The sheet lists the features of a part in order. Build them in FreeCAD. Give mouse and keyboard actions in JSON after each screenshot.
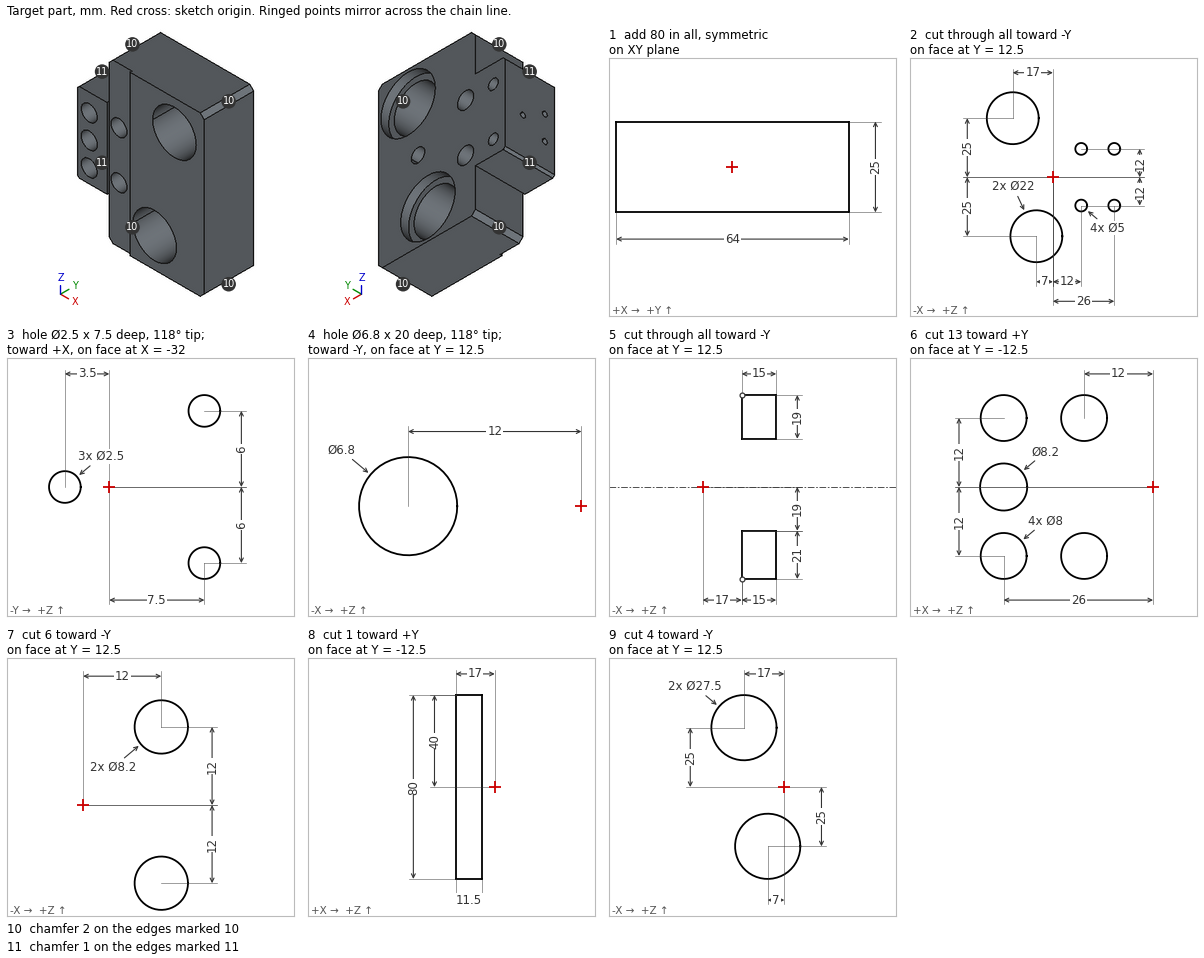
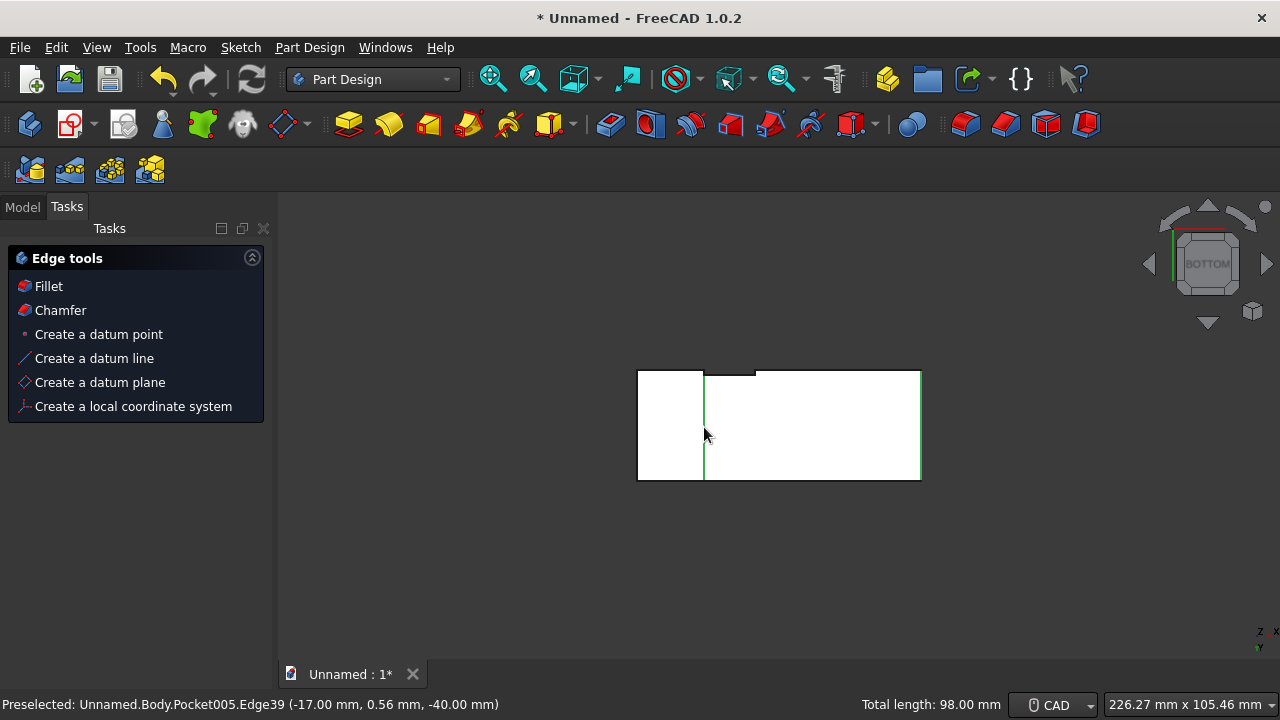
{"action": "left_click", "coordinate": [1006, 124]}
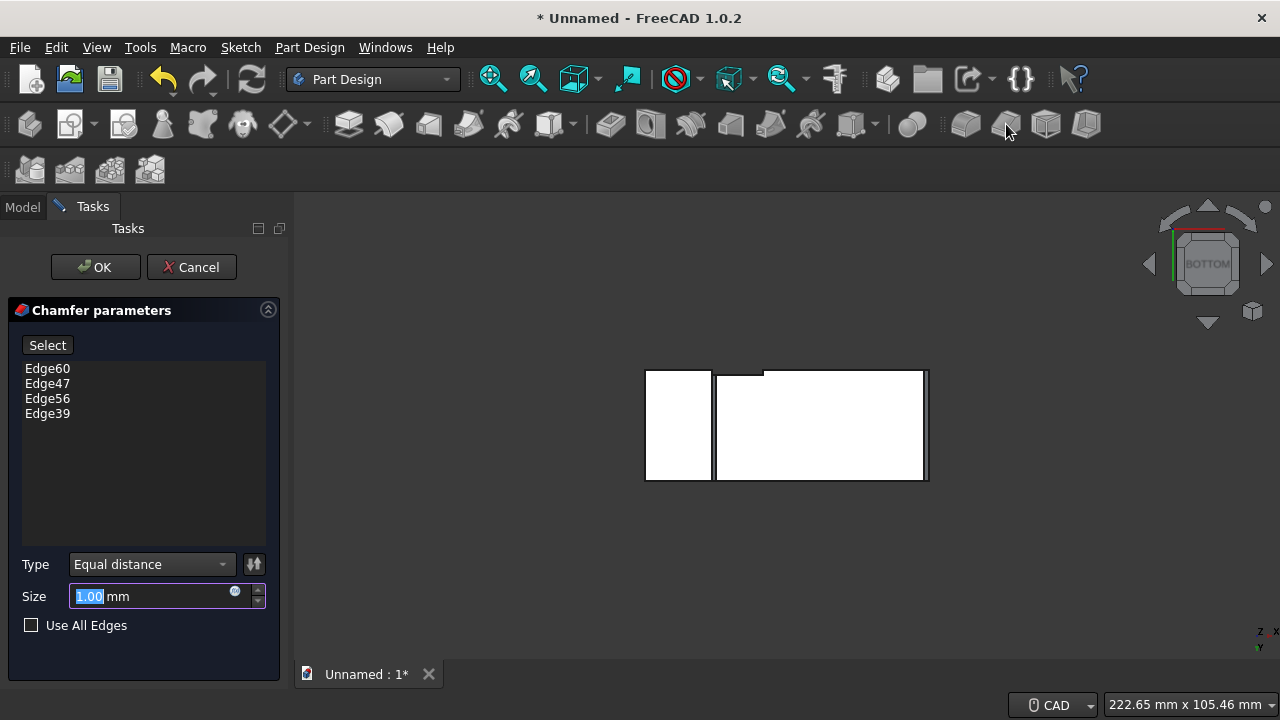
{"action": "type", "text": "2"}
{"action": "key", "text": "Tab"}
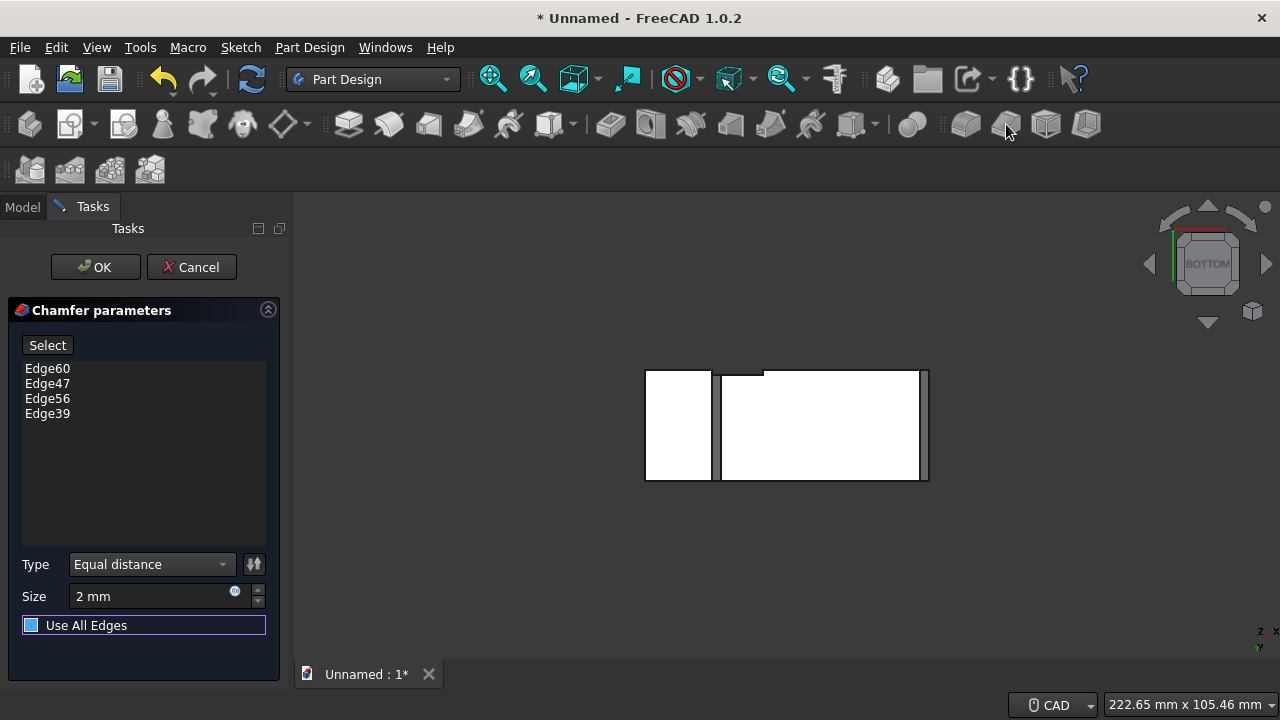
{"action": "left_click", "coordinate": [96, 267]}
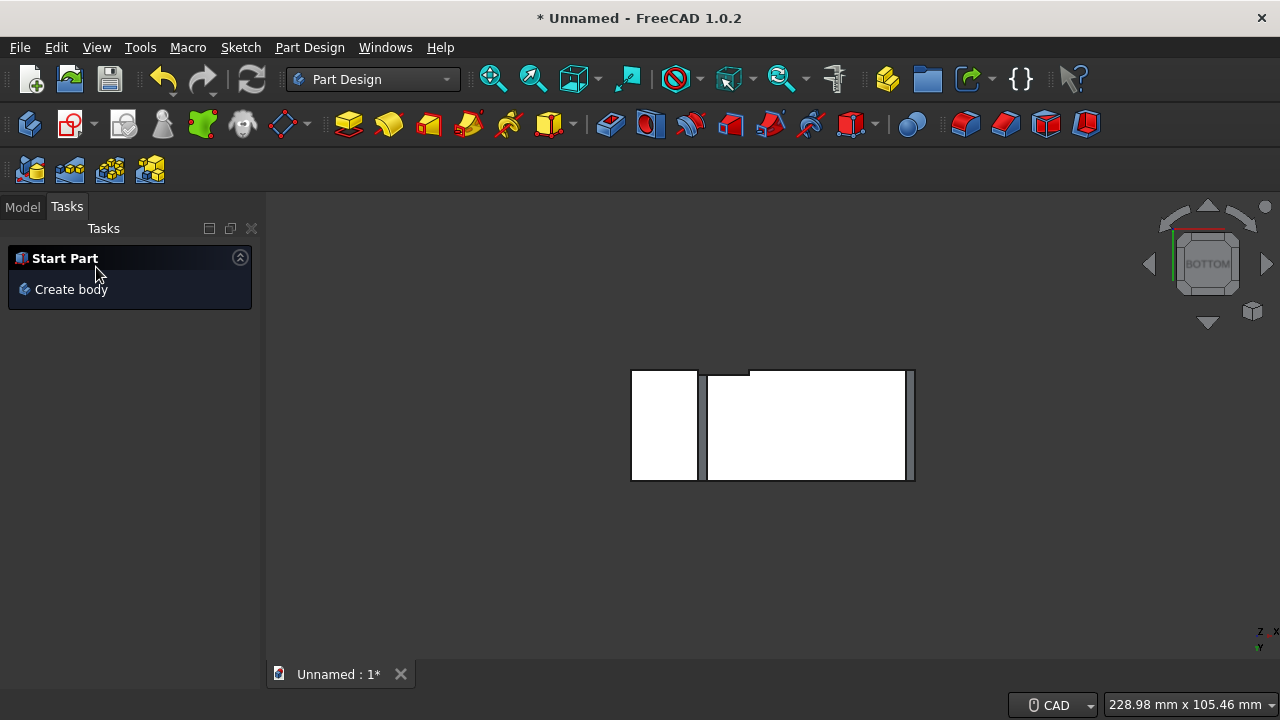
{"action": "left_click", "coordinate": [494, 80]}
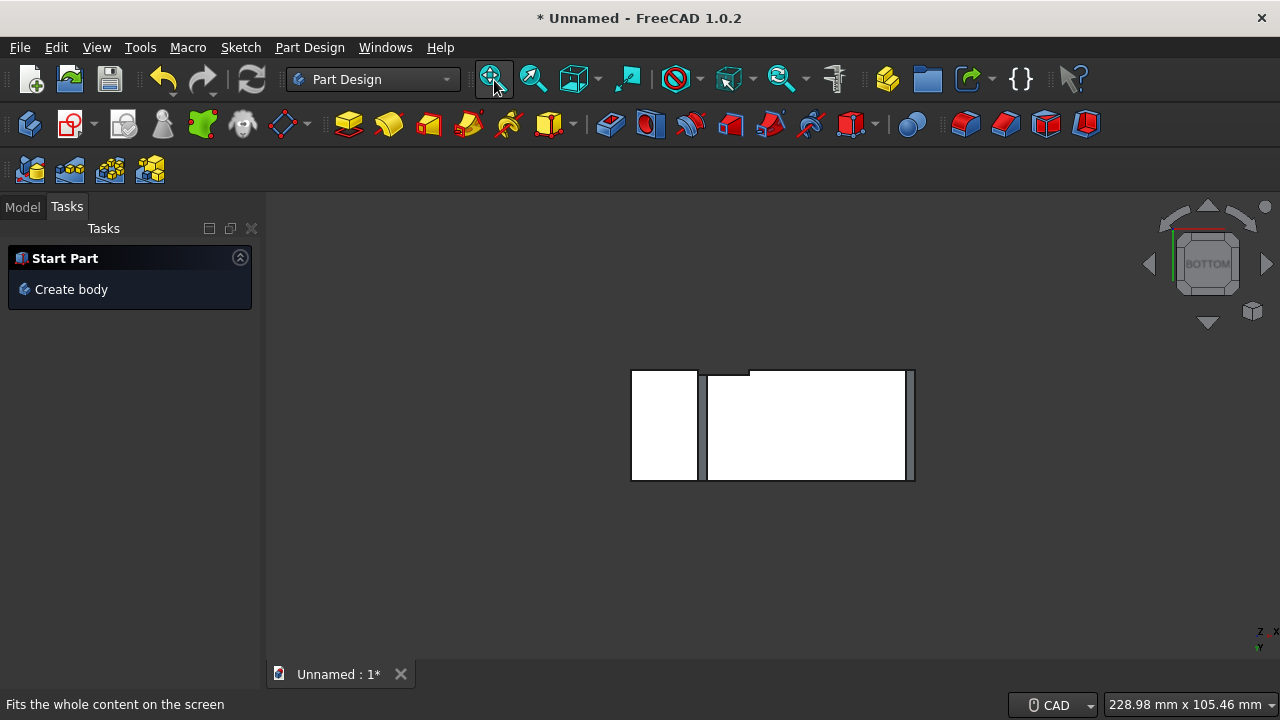
{"action": "left_click", "coordinate": [631, 424]}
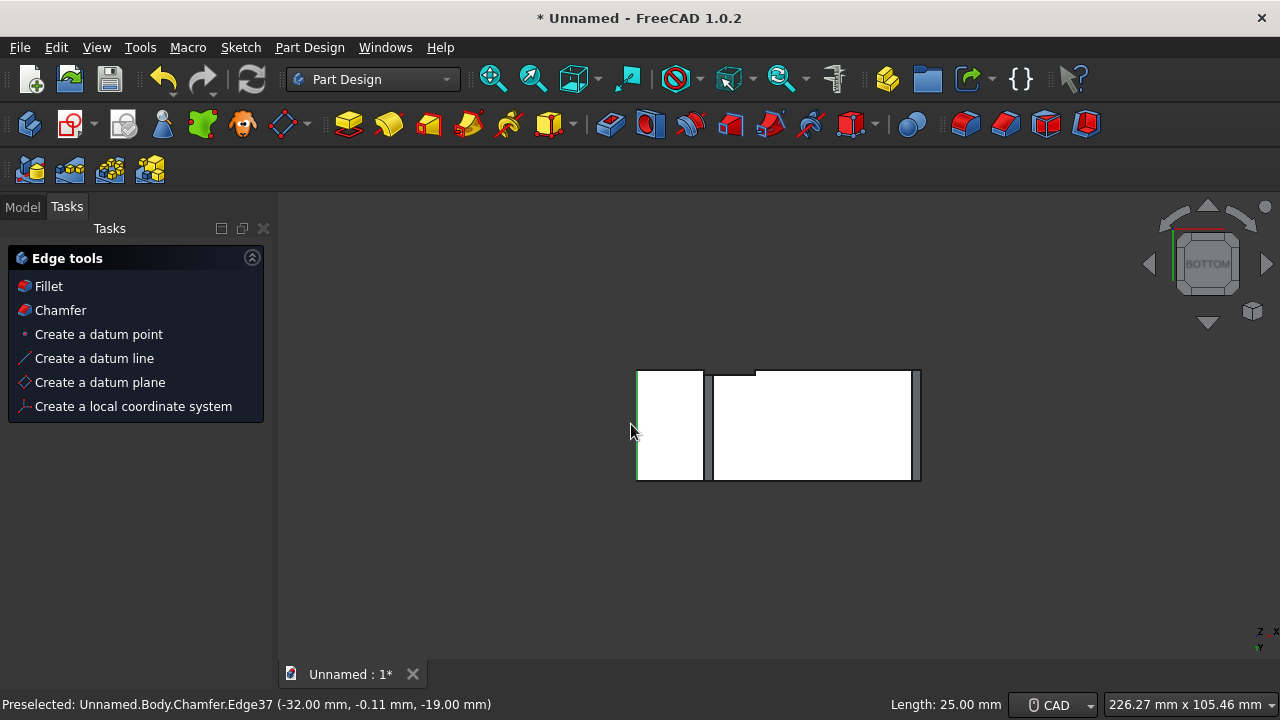
{"action": "key", "text": "0"}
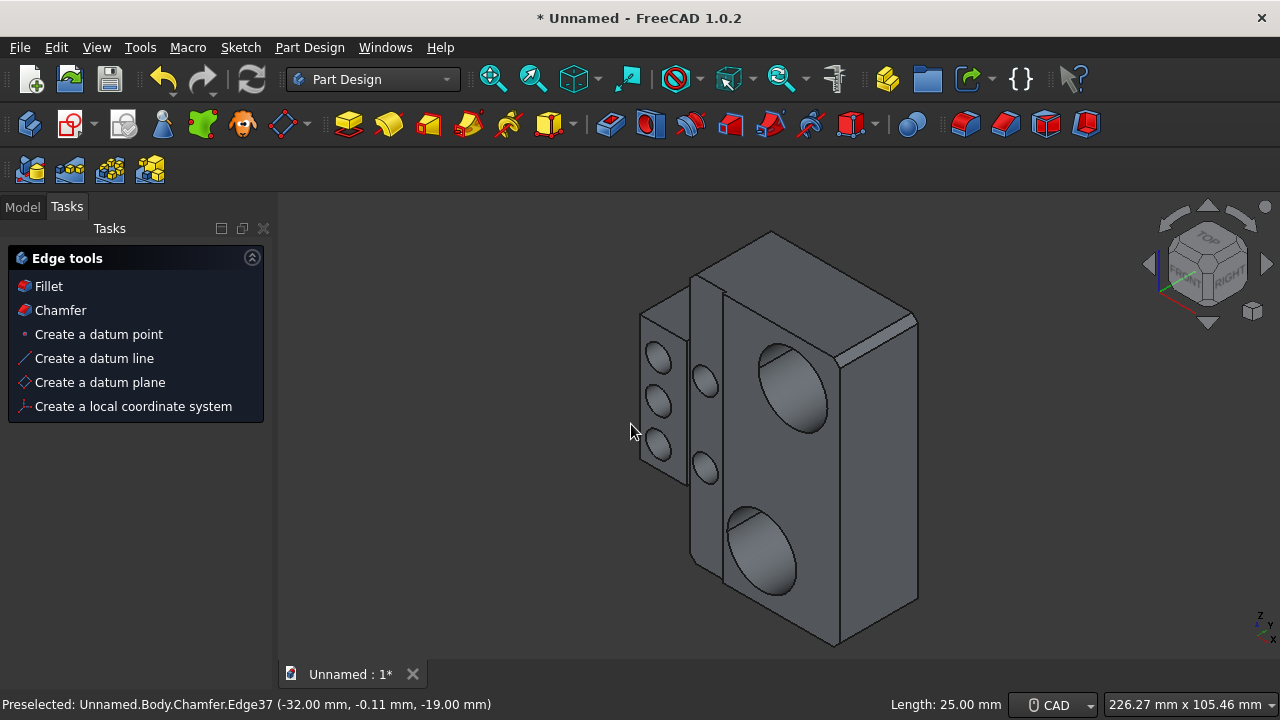
{"action": "key", "text": "2"}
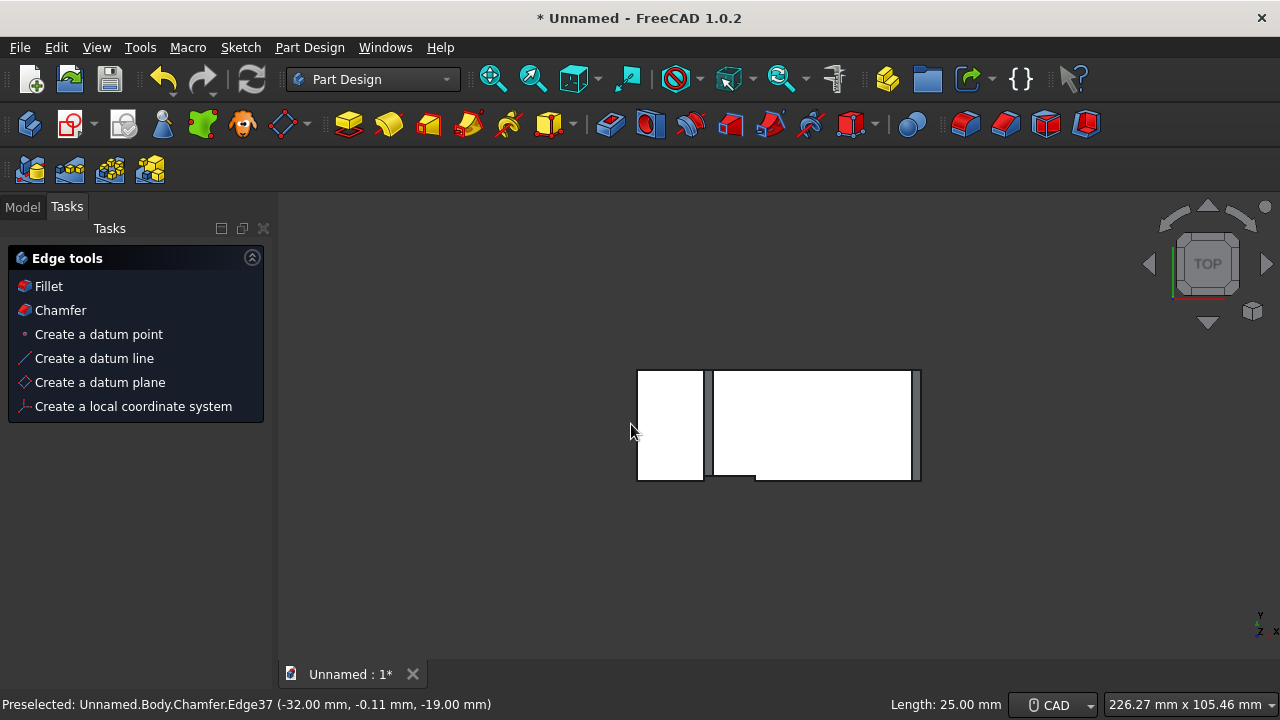
{"action": "left_click", "coordinate": [494, 80]}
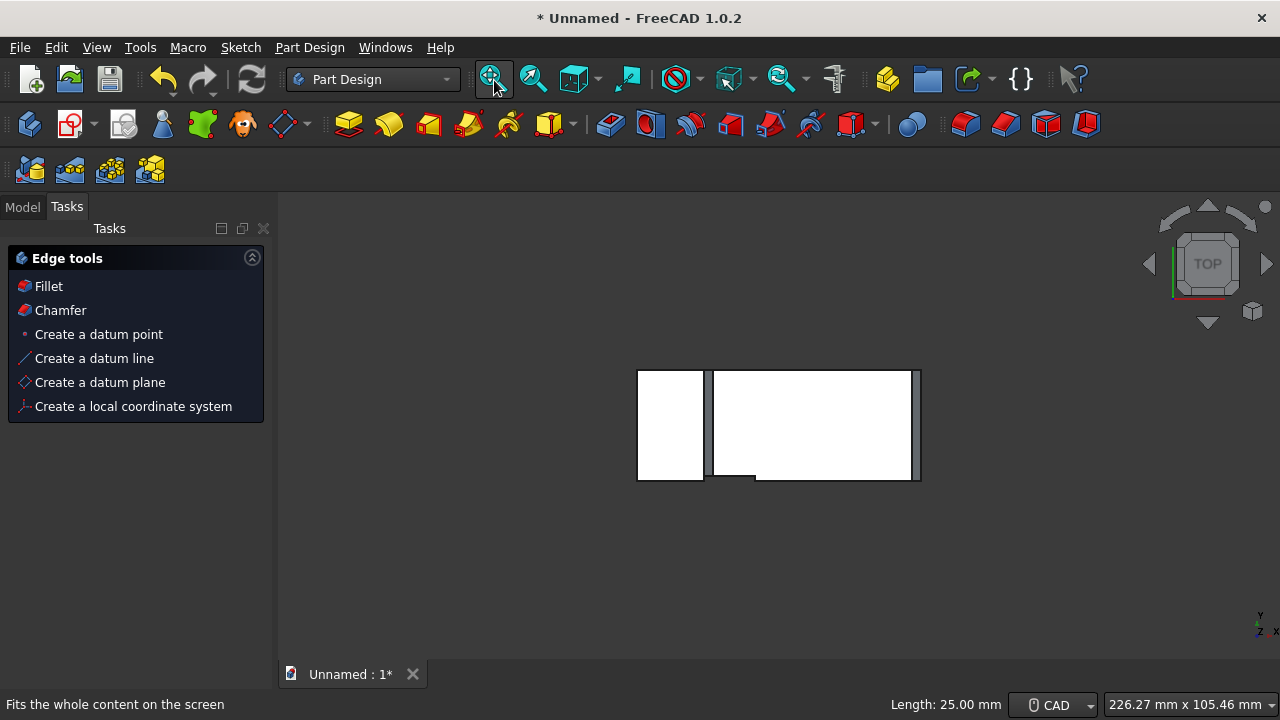
{"action": "left_click", "coordinate": [637, 424], "text": "ctrl"}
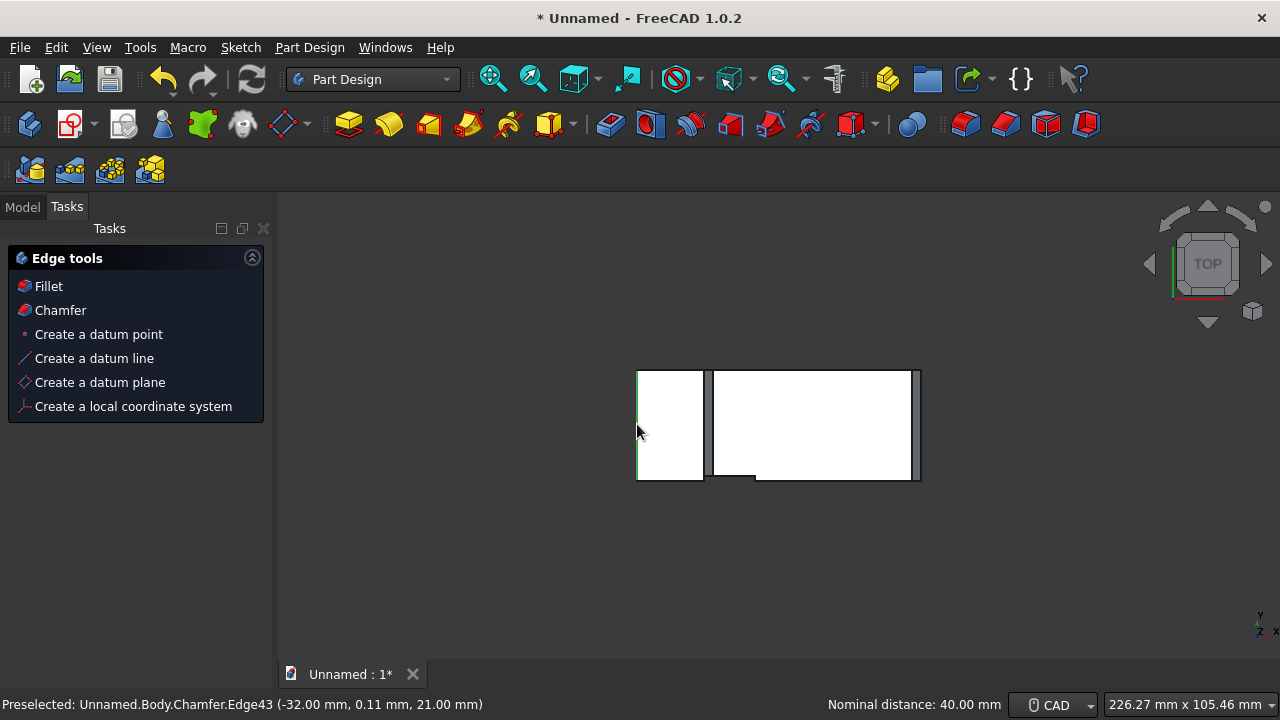
{"action": "left_click", "coordinate": [1006, 124]}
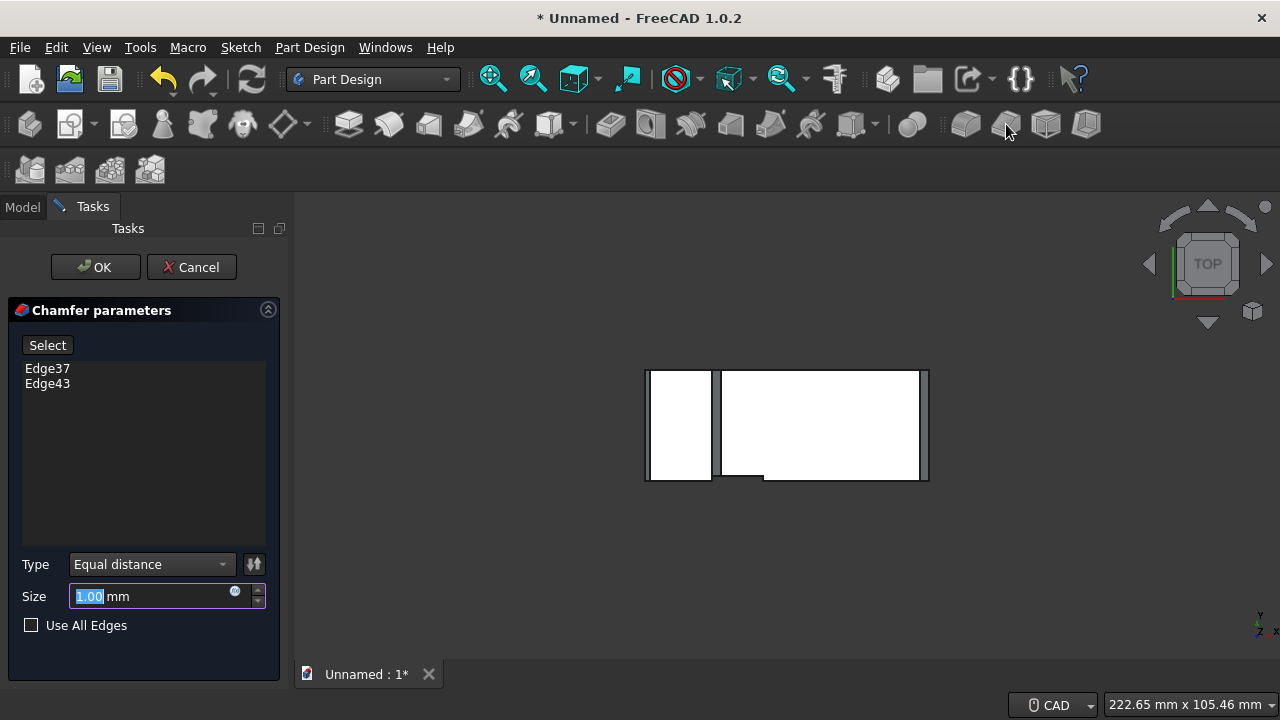
{"action": "type", "text": "1"}
{"action": "key", "text": "Tab"}